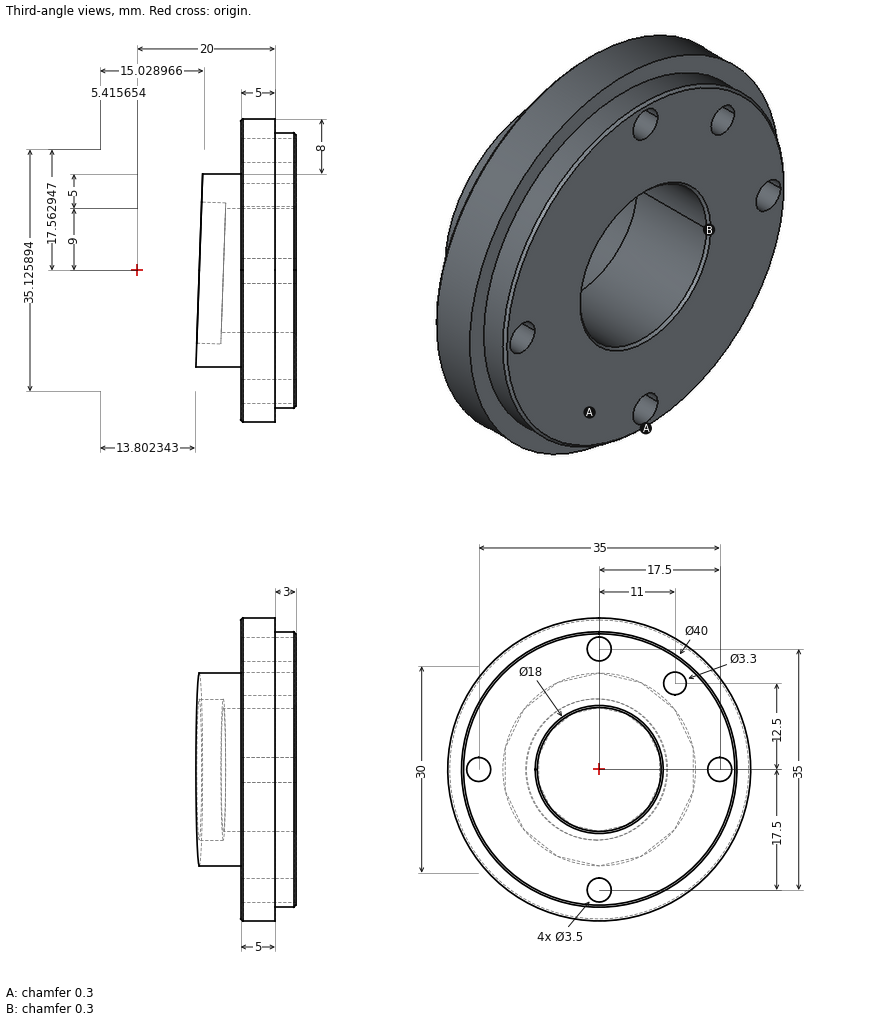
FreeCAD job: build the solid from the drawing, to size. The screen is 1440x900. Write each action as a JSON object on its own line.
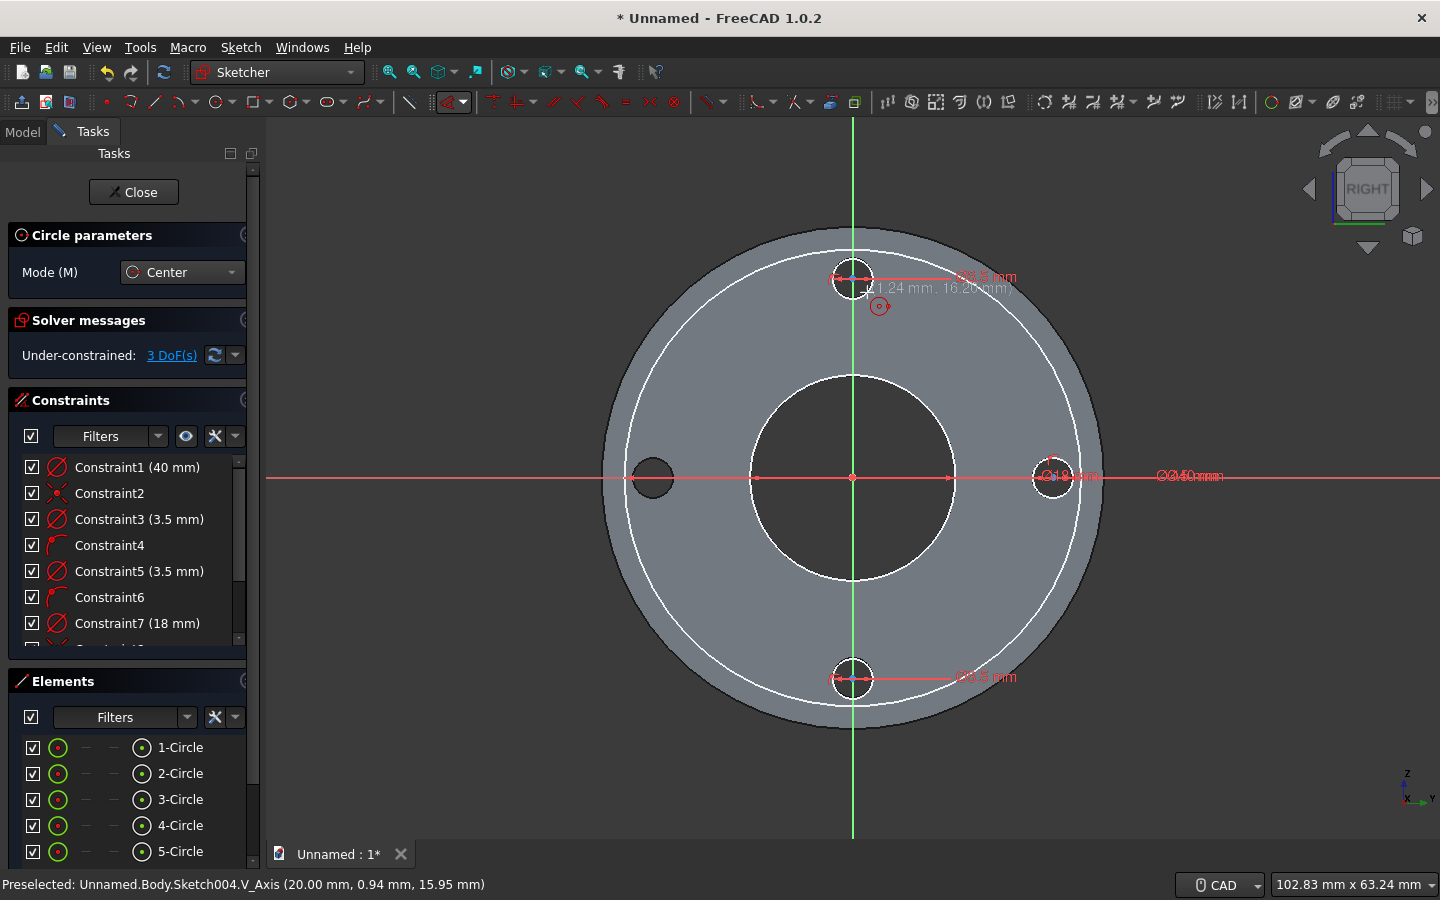
{"action": "left_click", "coordinate": [653, 478]}
{"action": "mouse_move", "coordinate": [667, 464]}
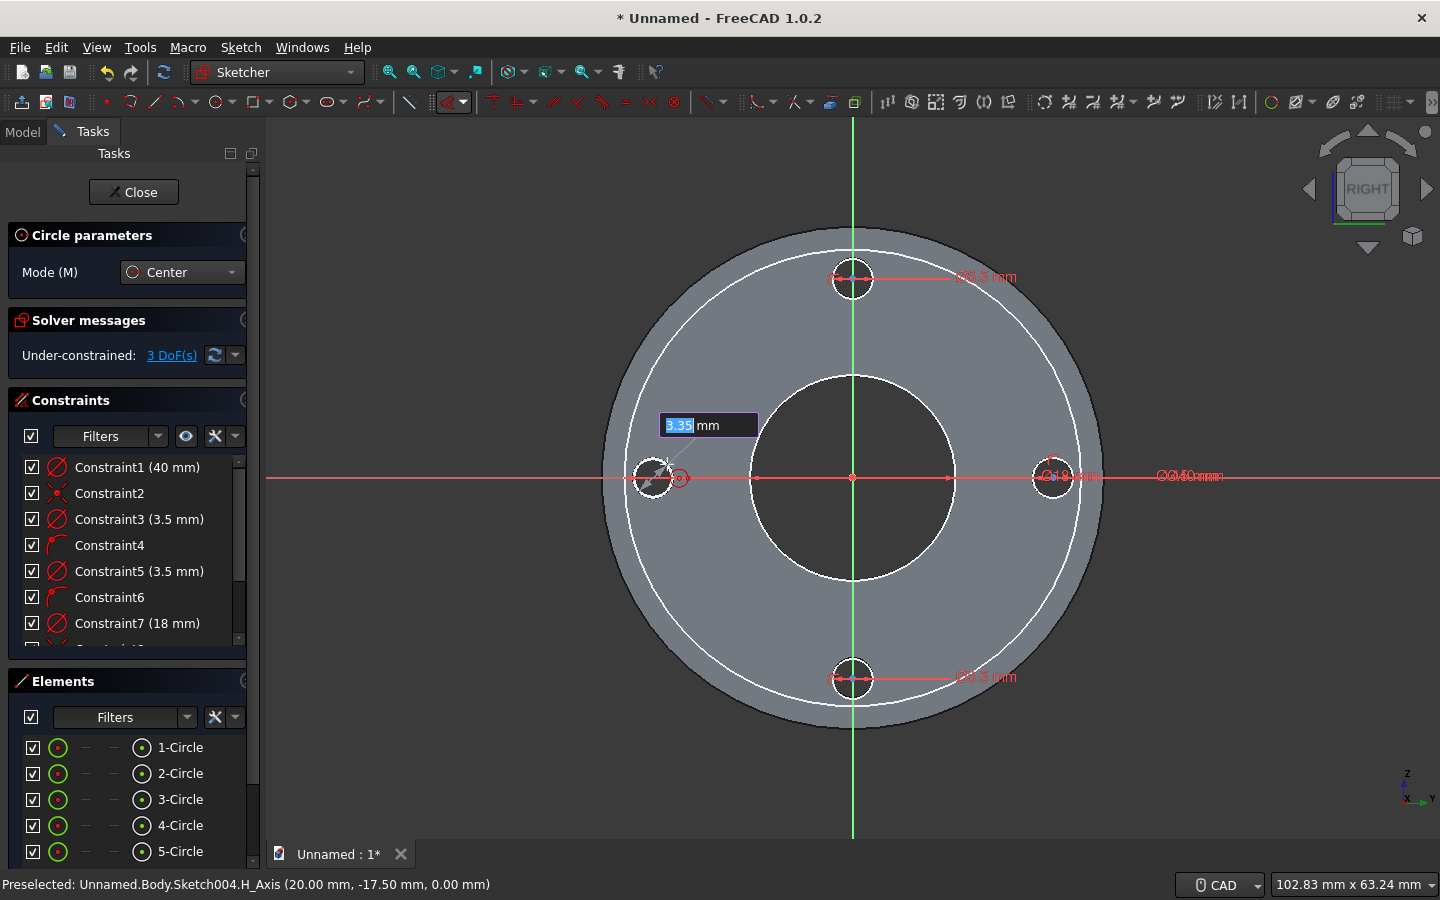
{"action": "type", "text": "3.5"}
{"action": "key", "text": "Return"}
{"action": "key", "text": "Escape"}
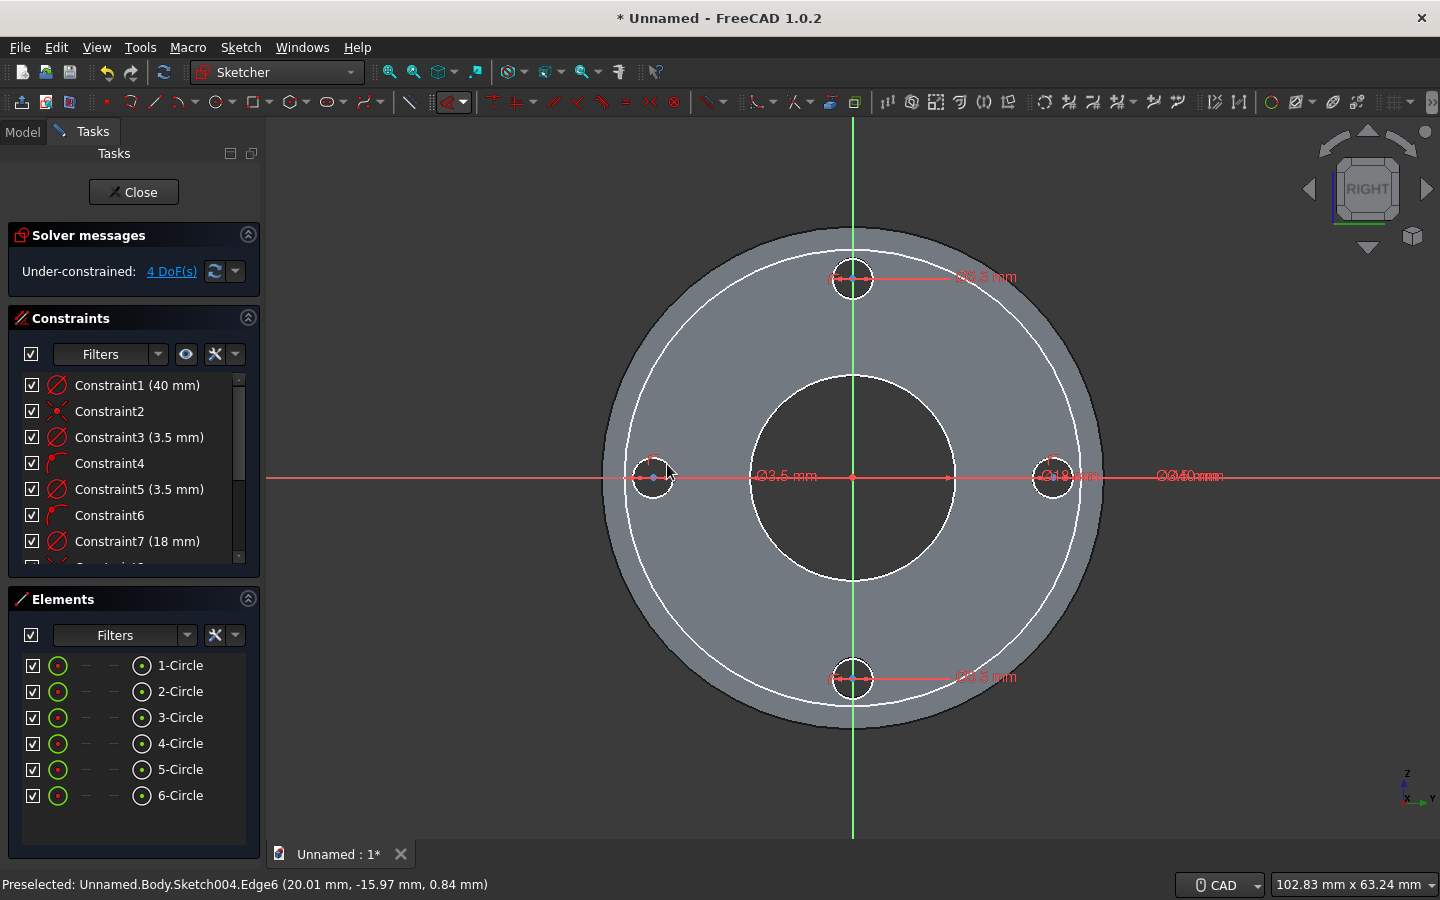
{"action": "left_click", "coordinate": [853, 679]}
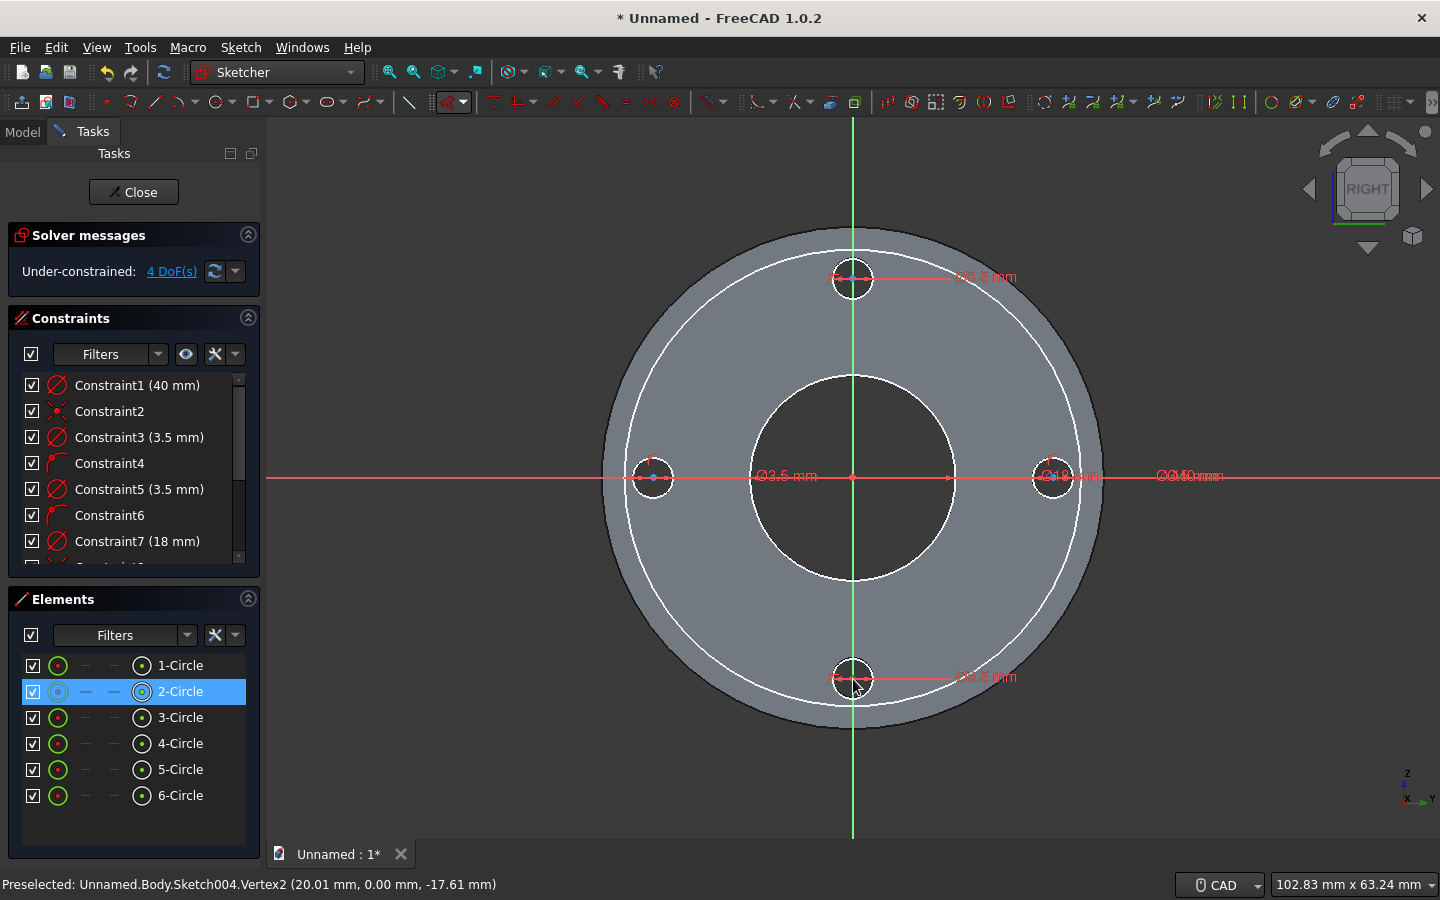
{"action": "left_click", "coordinate": [853, 279]}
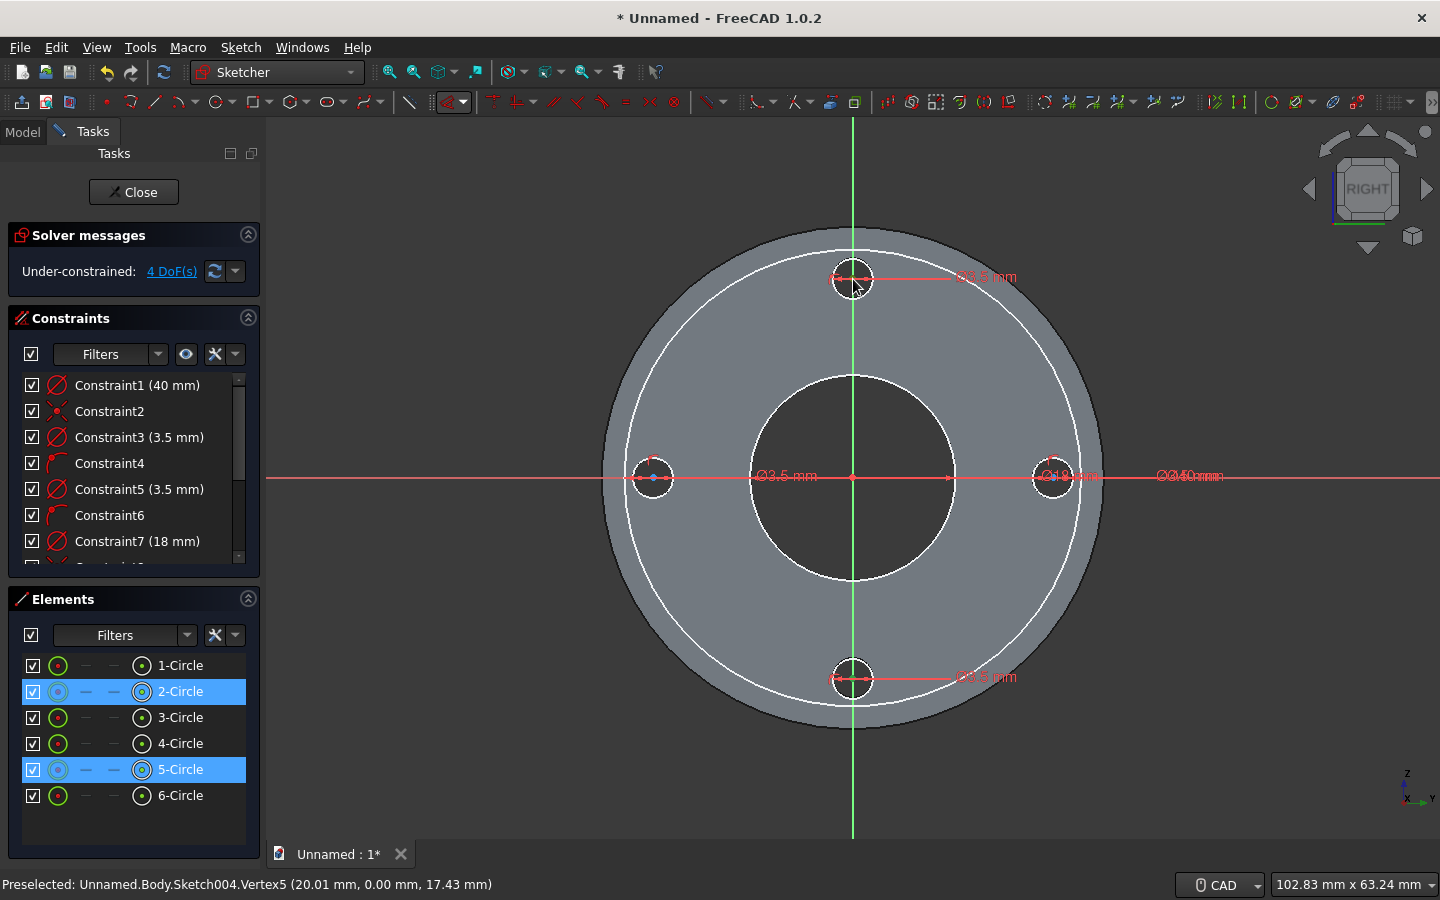
{"action": "key", "text": "i"}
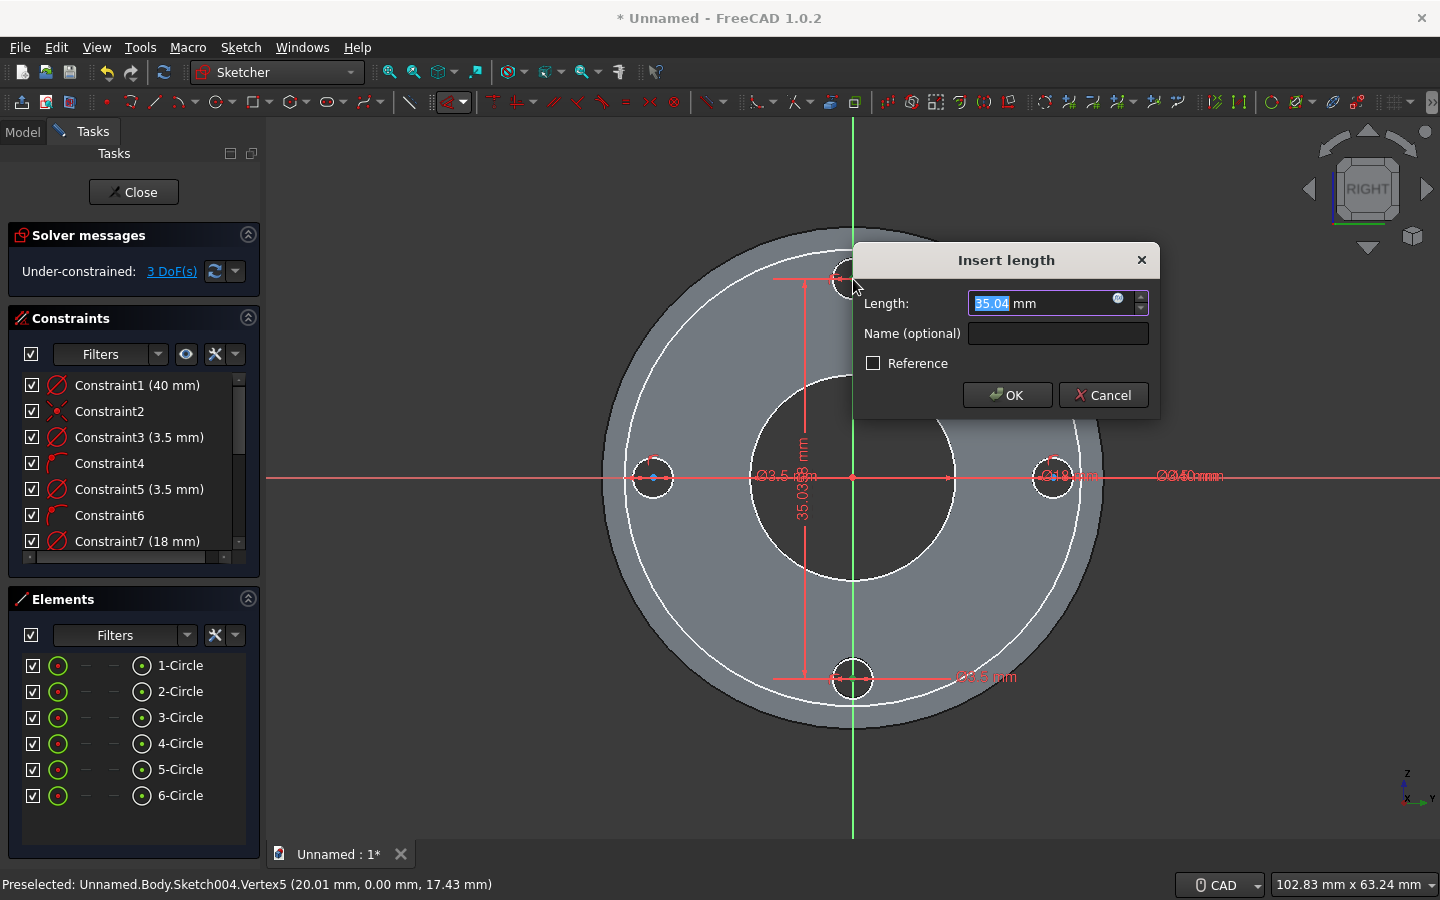
{"action": "type", "text": "35"}
{"action": "key", "text": "Return"}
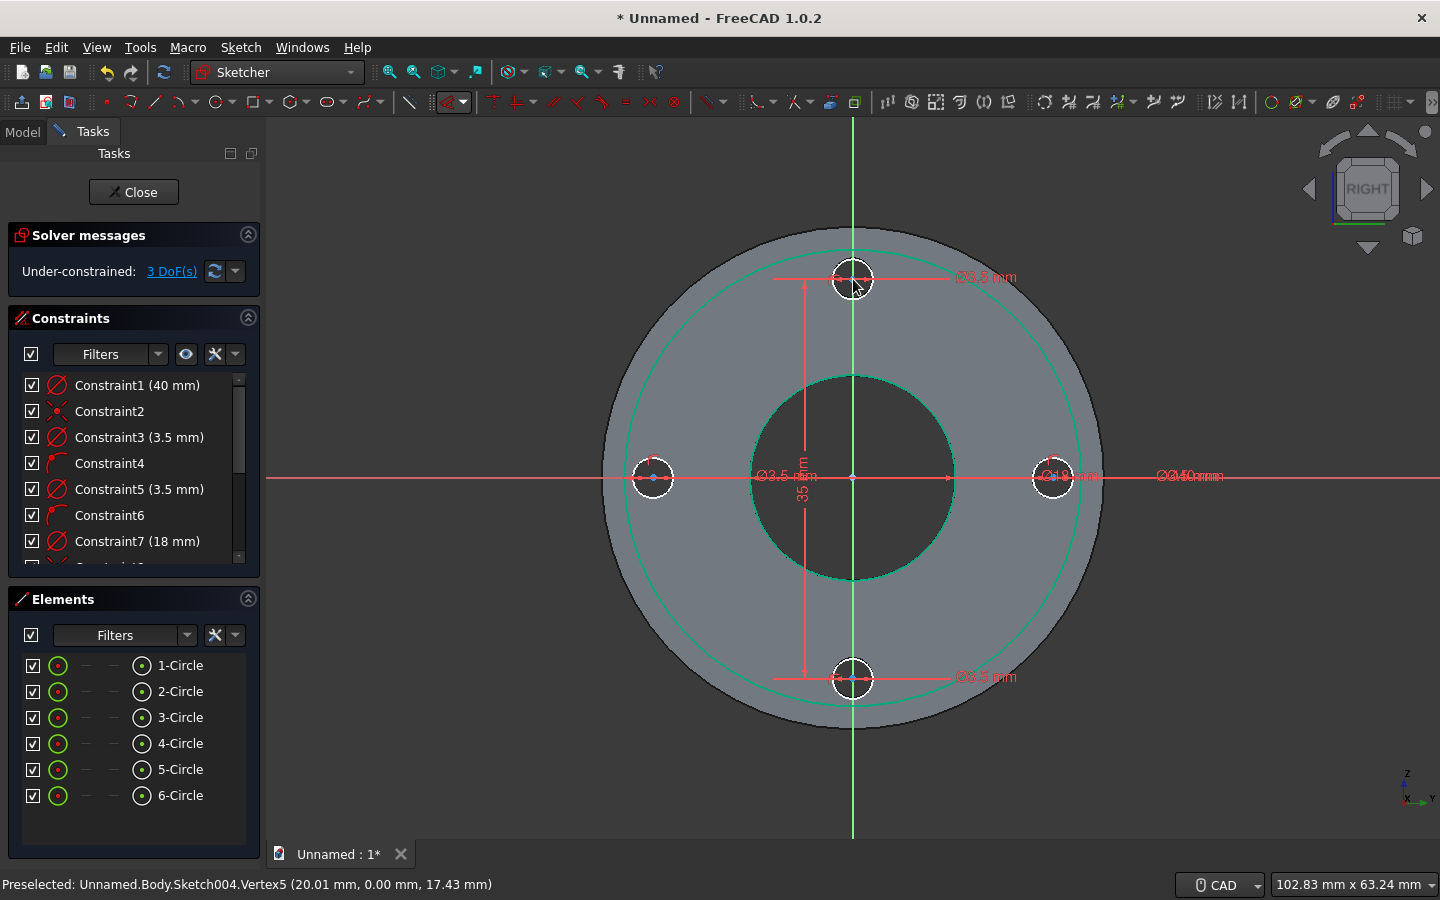
{"action": "left_click", "coordinate": [1053, 478]}